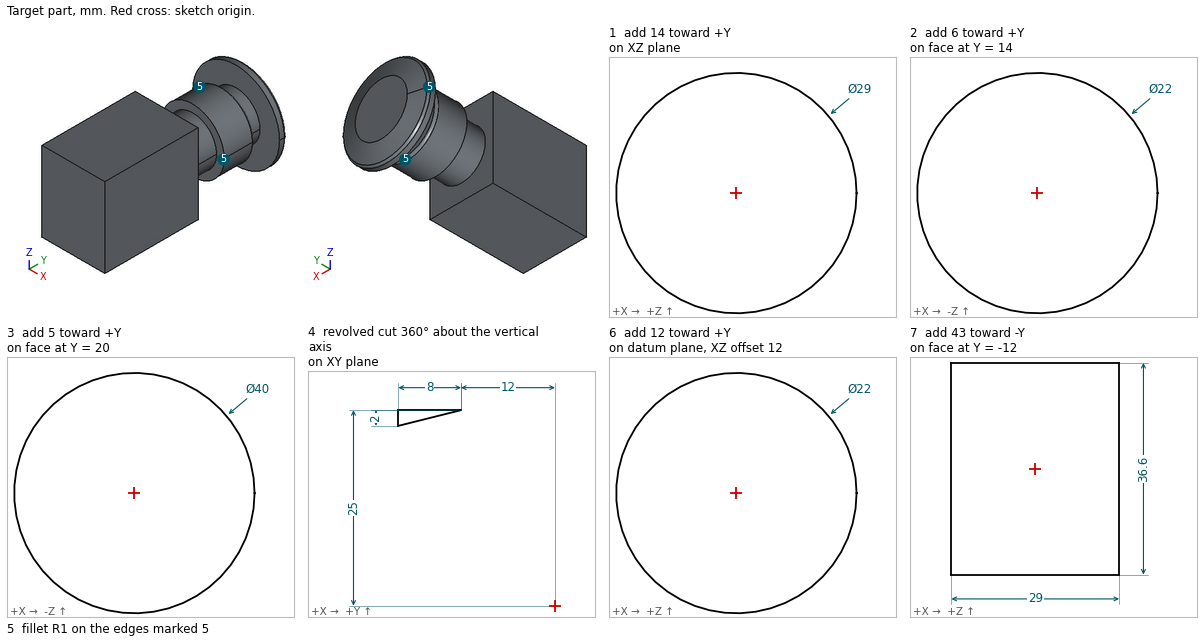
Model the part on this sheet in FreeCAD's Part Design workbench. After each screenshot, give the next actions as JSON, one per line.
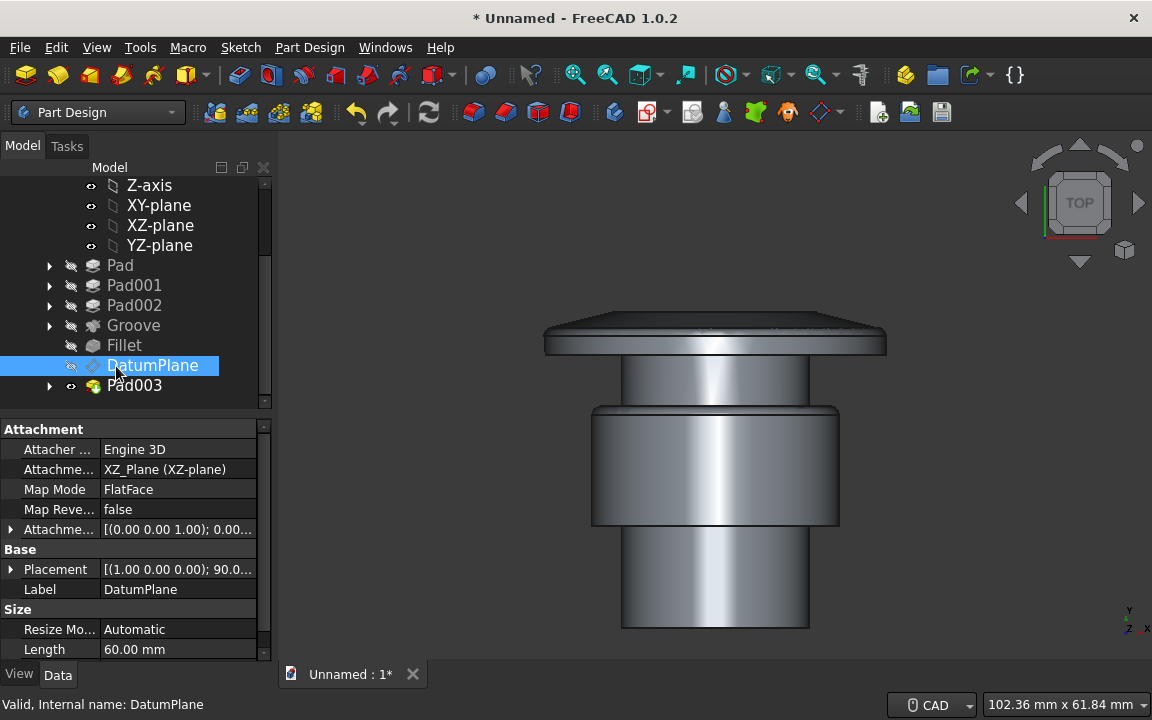
{"action": "key", "text": "0"}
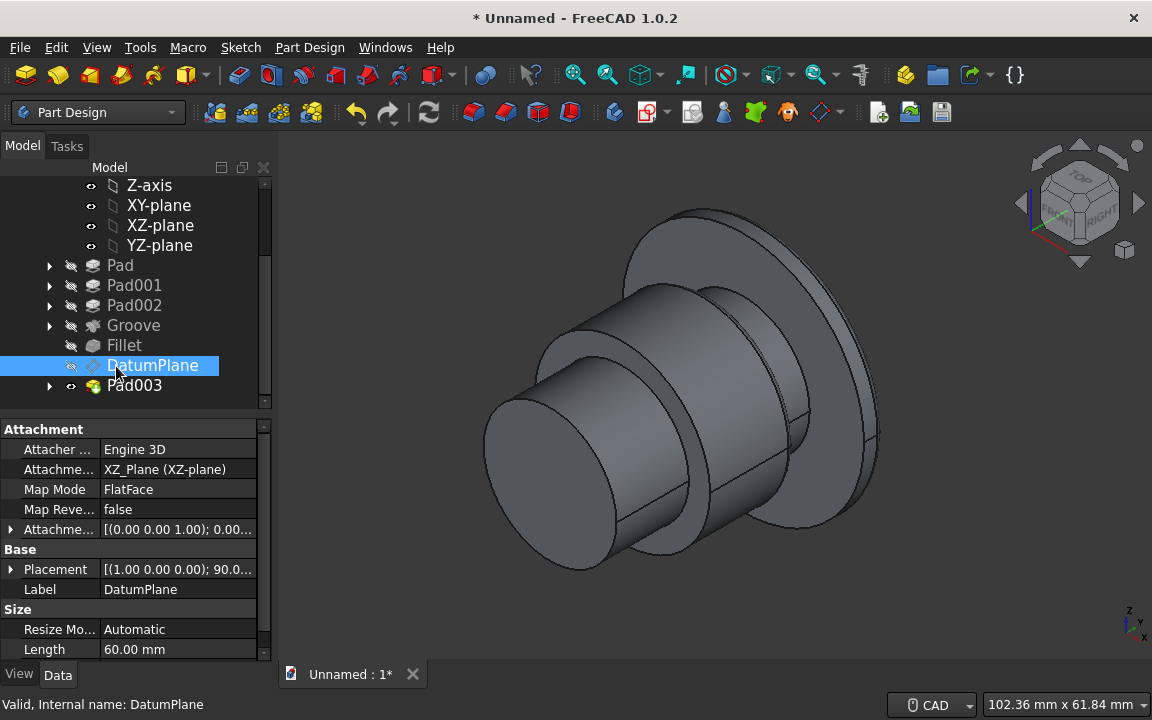
{"action": "left_click", "coordinate": [576, 76]}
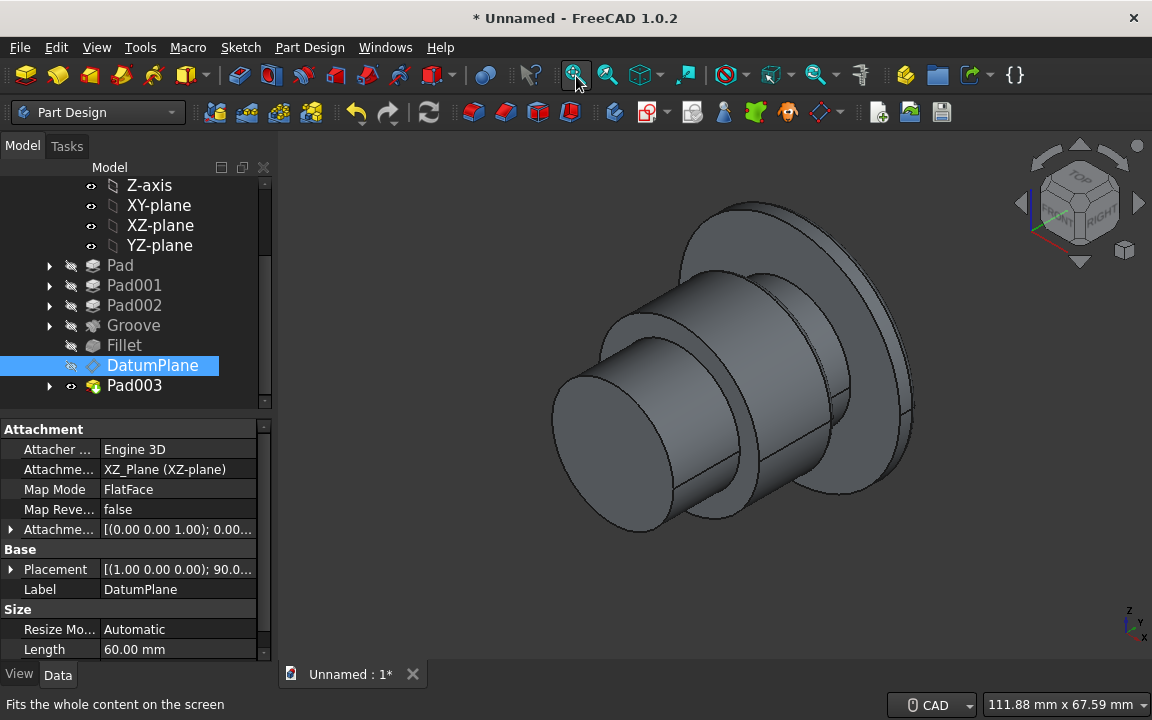
{"action": "left_click", "coordinate": [613, 453]}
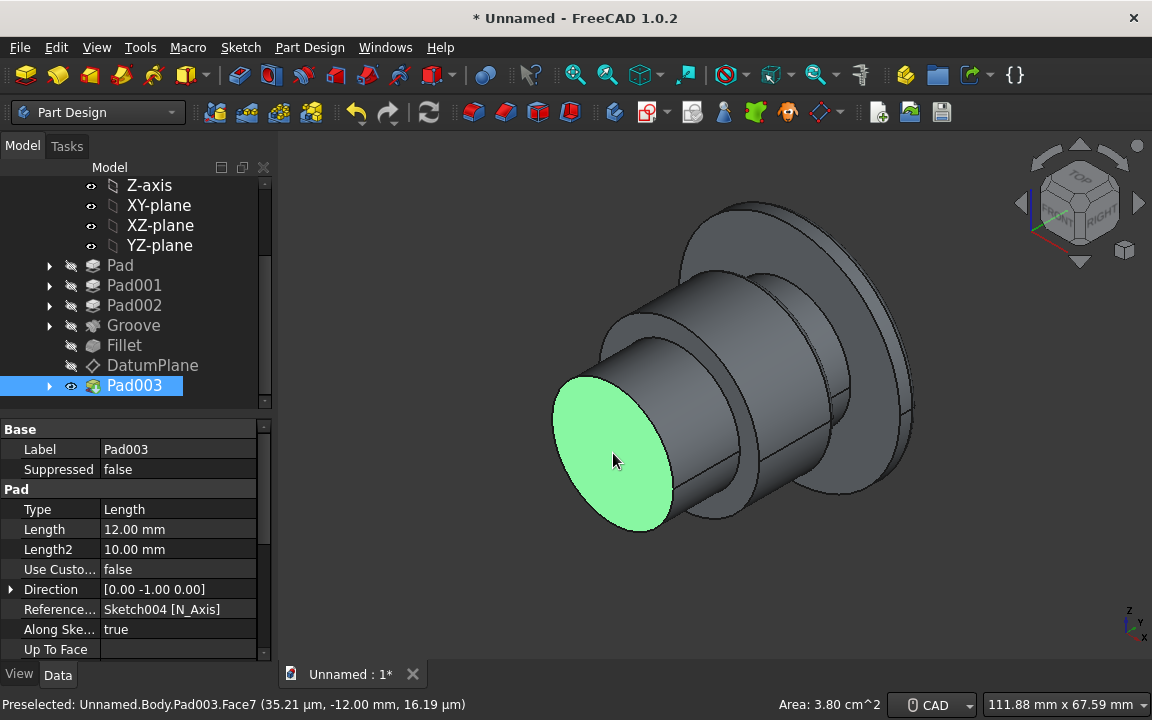
{"action": "left_click", "coordinate": [648, 112]}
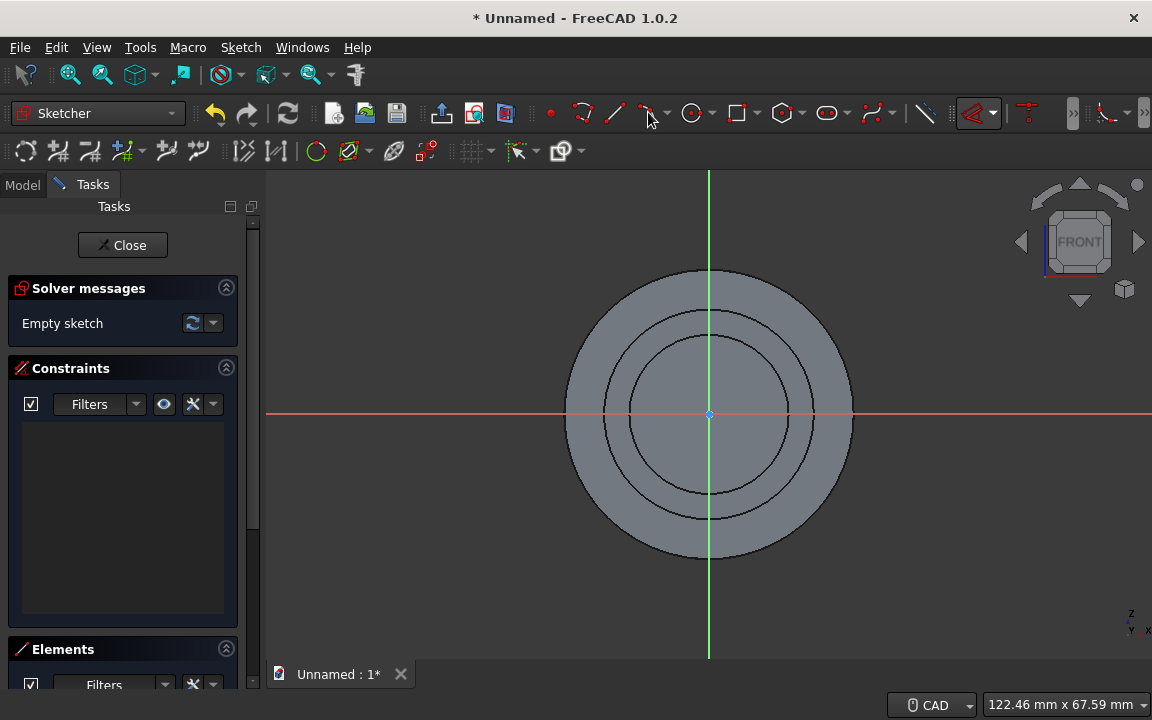
{"action": "key", "text": "g v"}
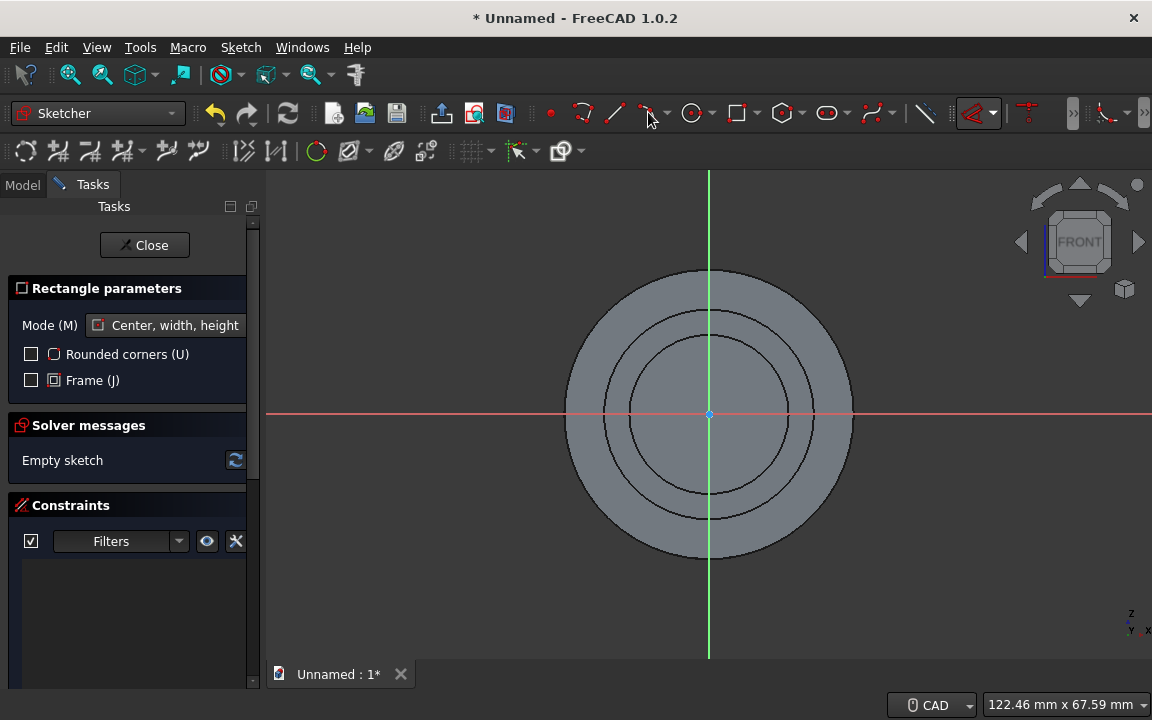
{"action": "left_click", "coordinate": [709, 414]}
{"action": "left_click", "coordinate": [814, 282]}
{"action": "key", "text": "Escape"}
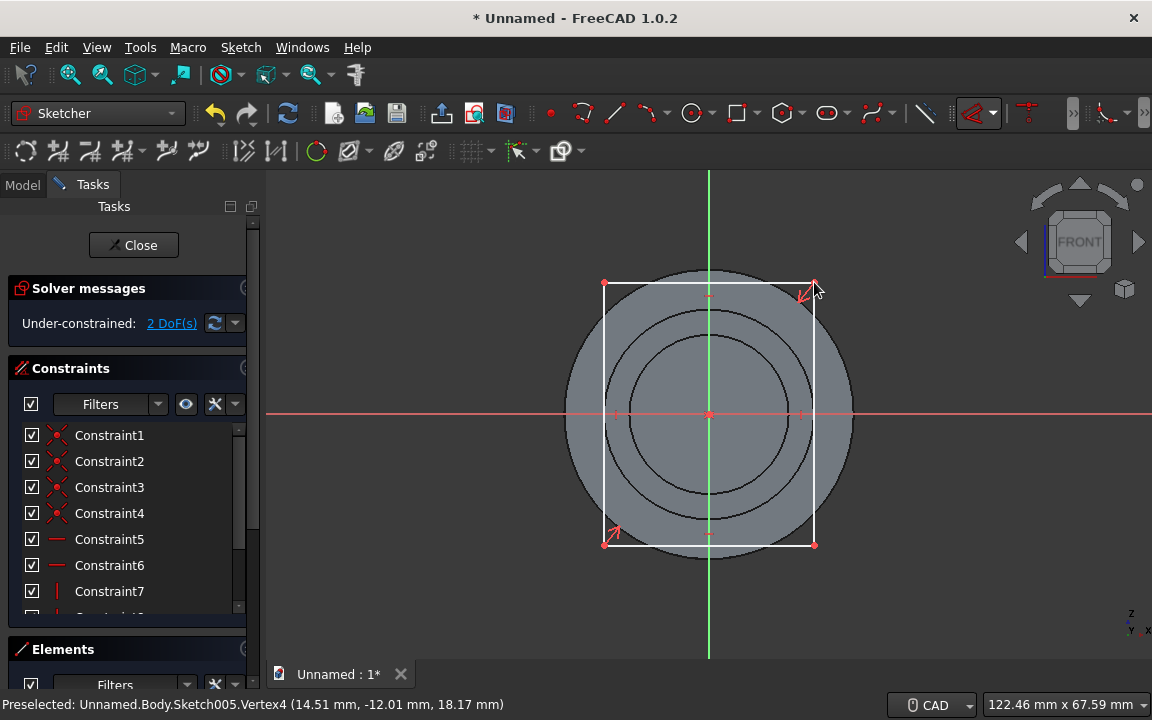
{"action": "left_click", "coordinate": [667, 546]}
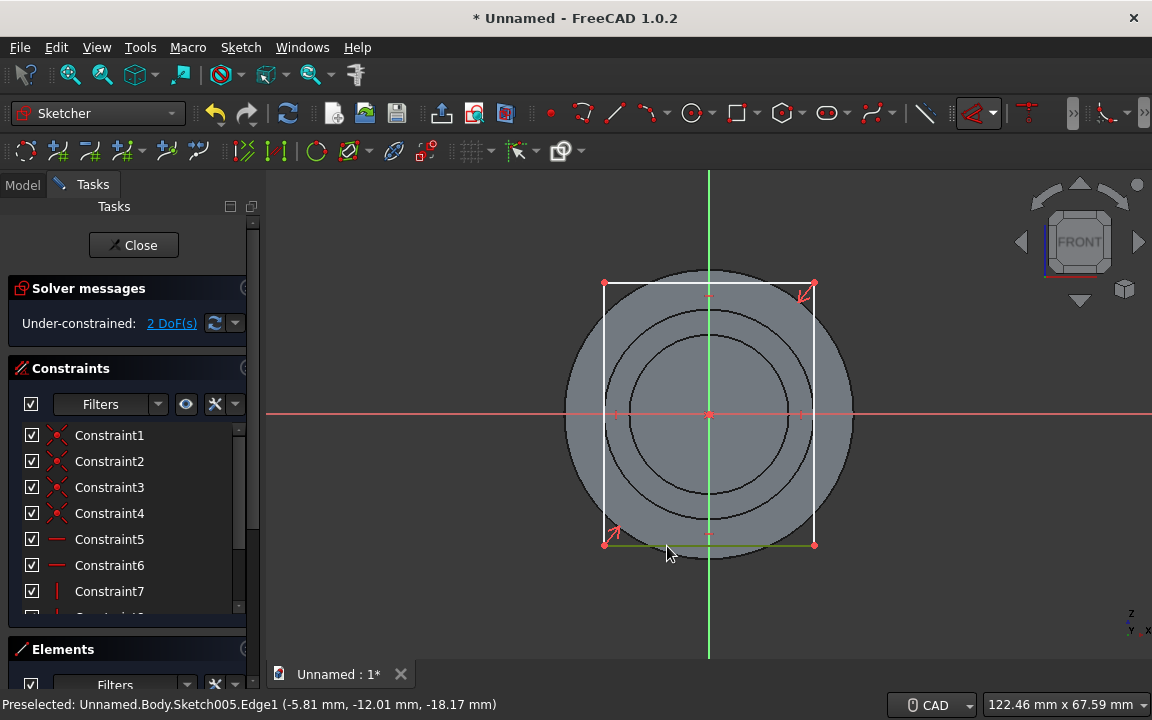
{"action": "key", "text": "l"}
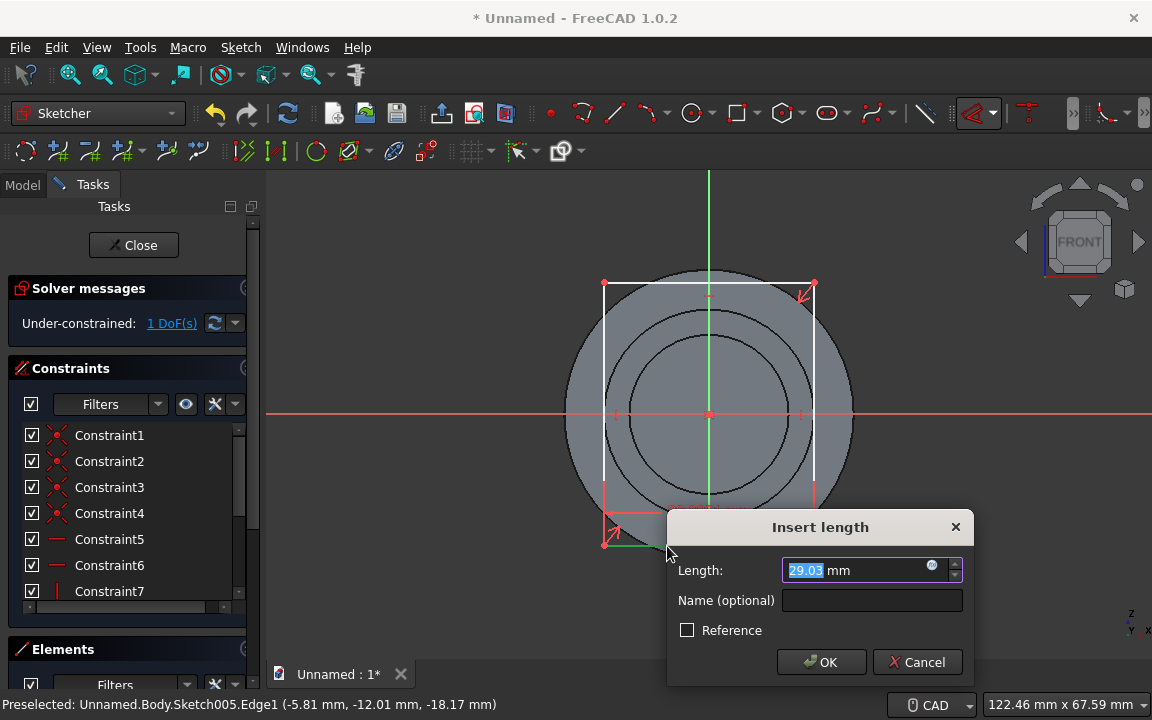
{"action": "type", "text": "29"}
{"action": "key", "text": "Return"}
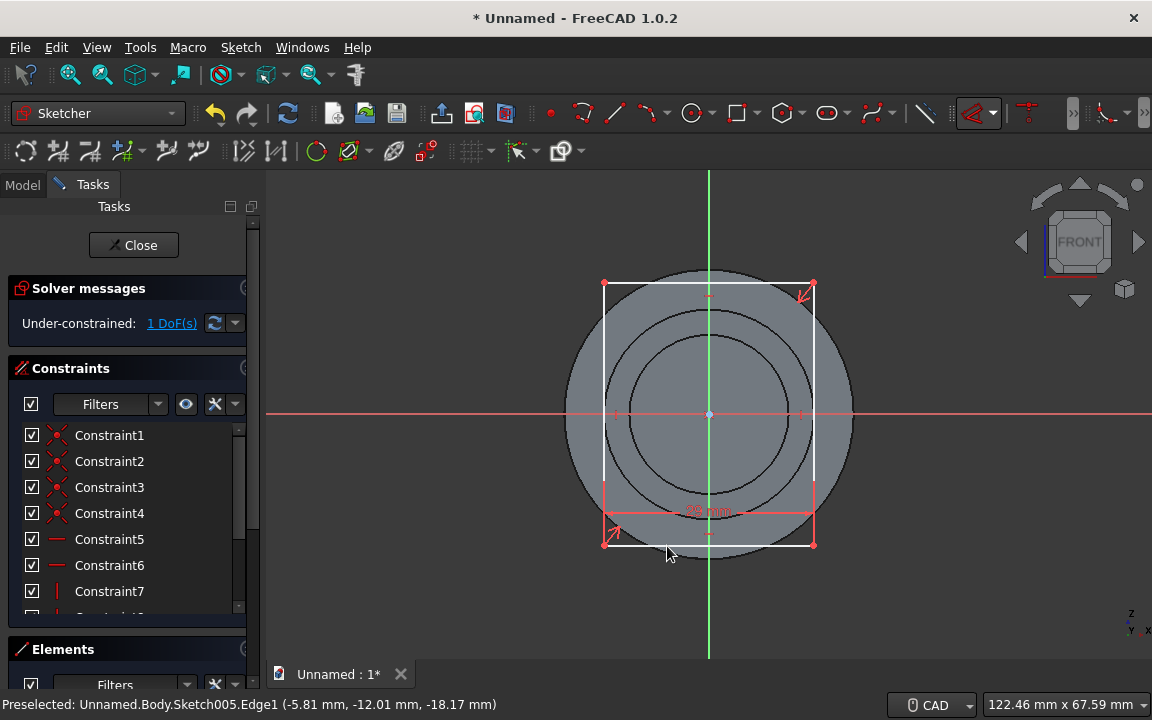
{"action": "left_click", "coordinate": [814, 467]}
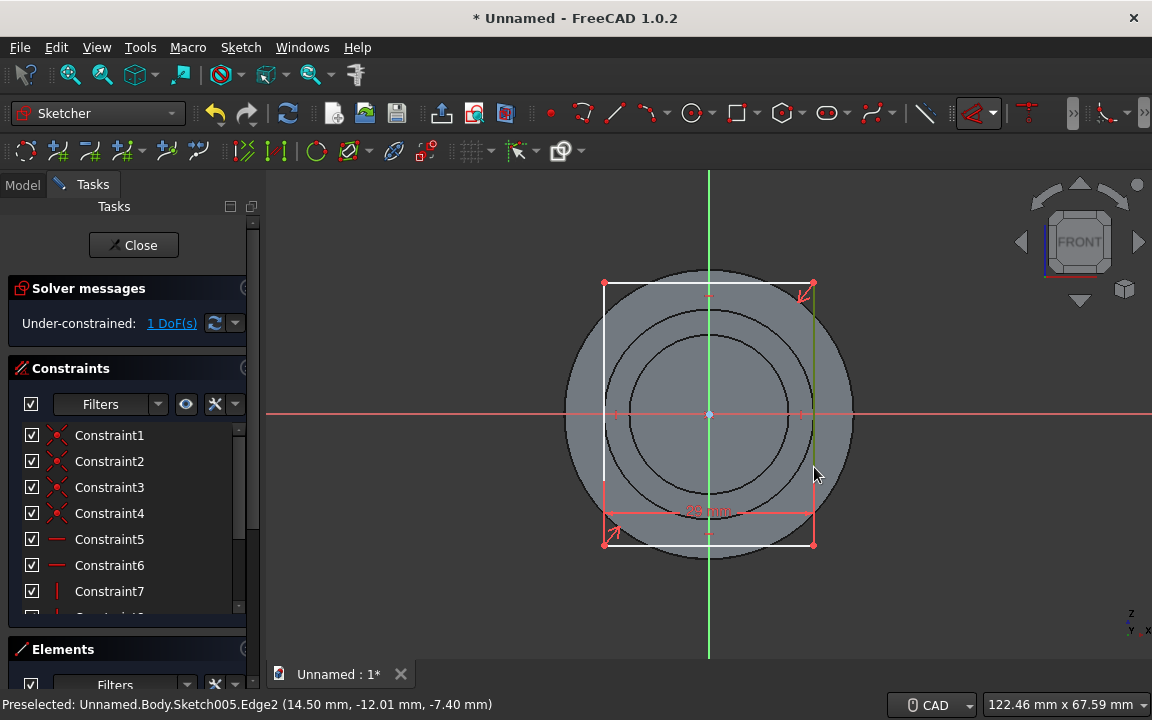
{"action": "left_click", "coordinate": [996, 114]}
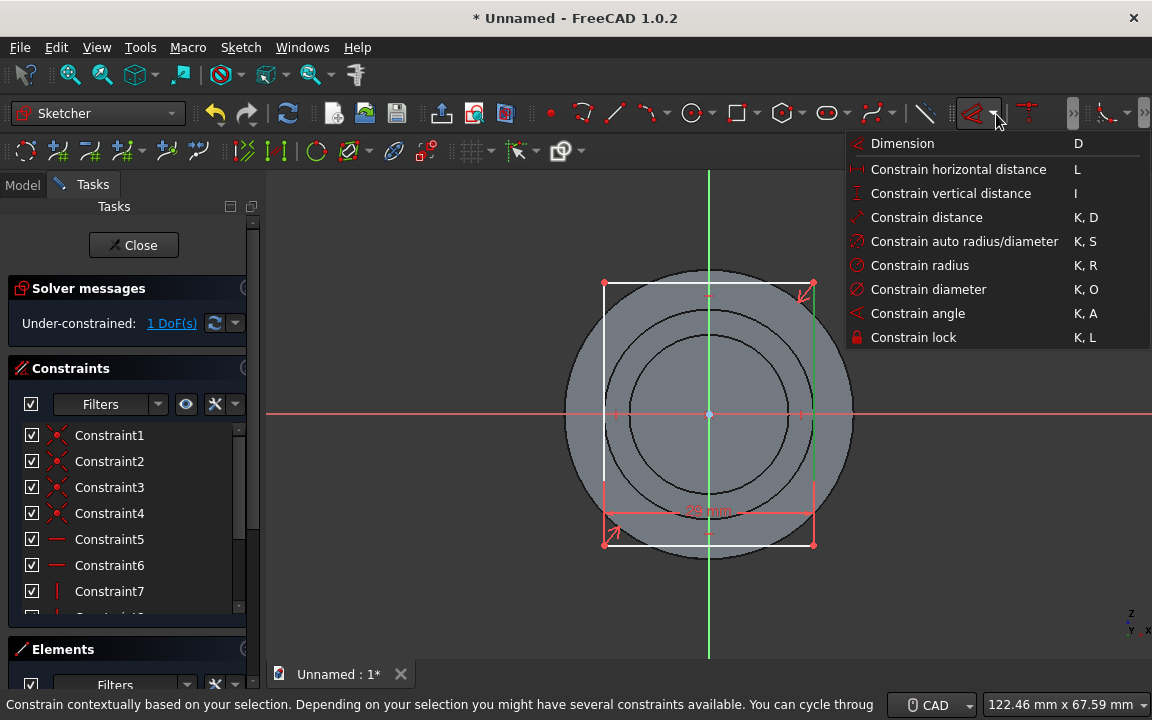
{"action": "left_click", "coordinate": [998, 193]}